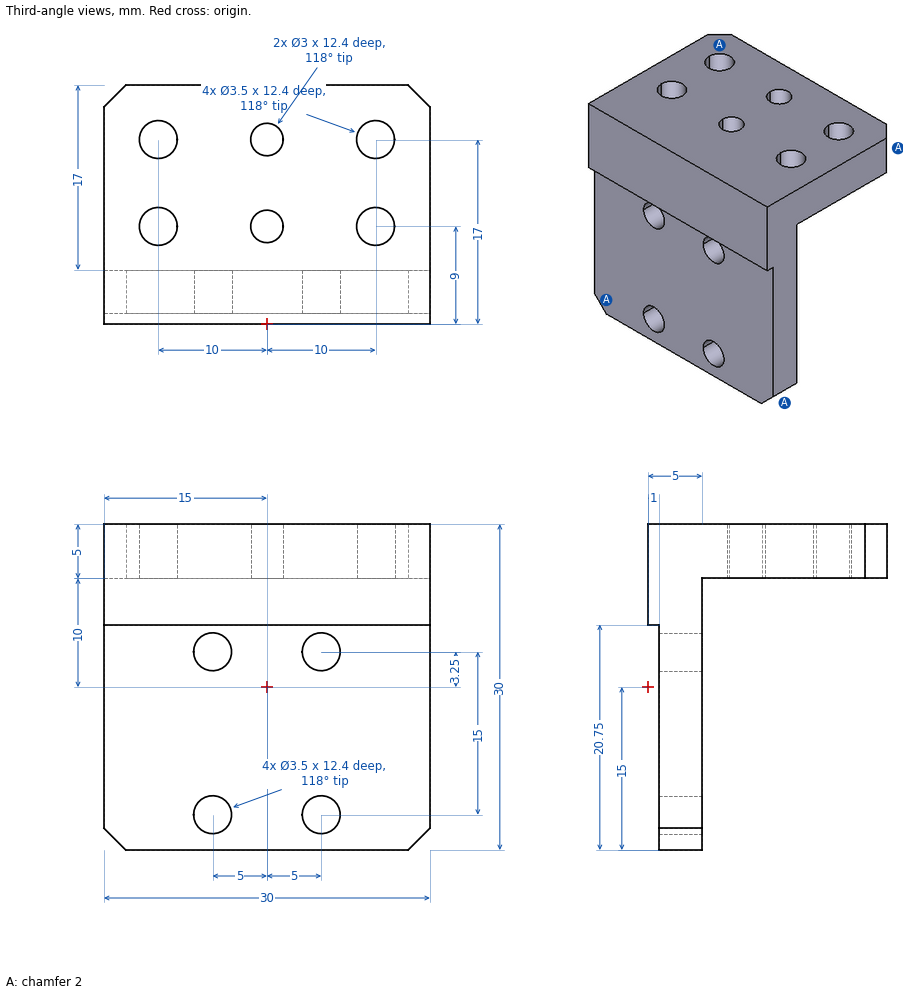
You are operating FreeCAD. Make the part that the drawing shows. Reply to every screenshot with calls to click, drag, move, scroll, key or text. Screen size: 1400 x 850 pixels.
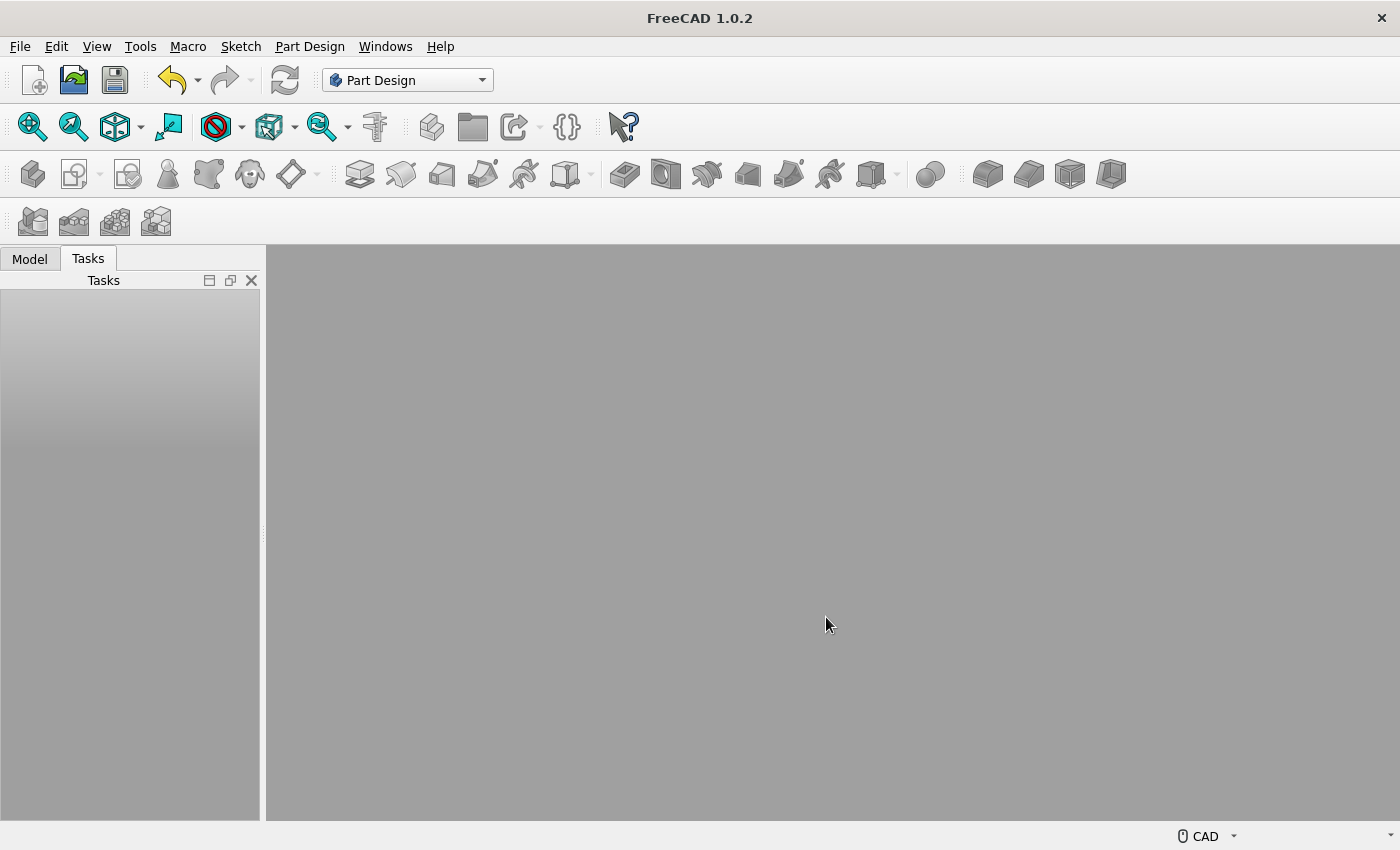
key(ctrl+n)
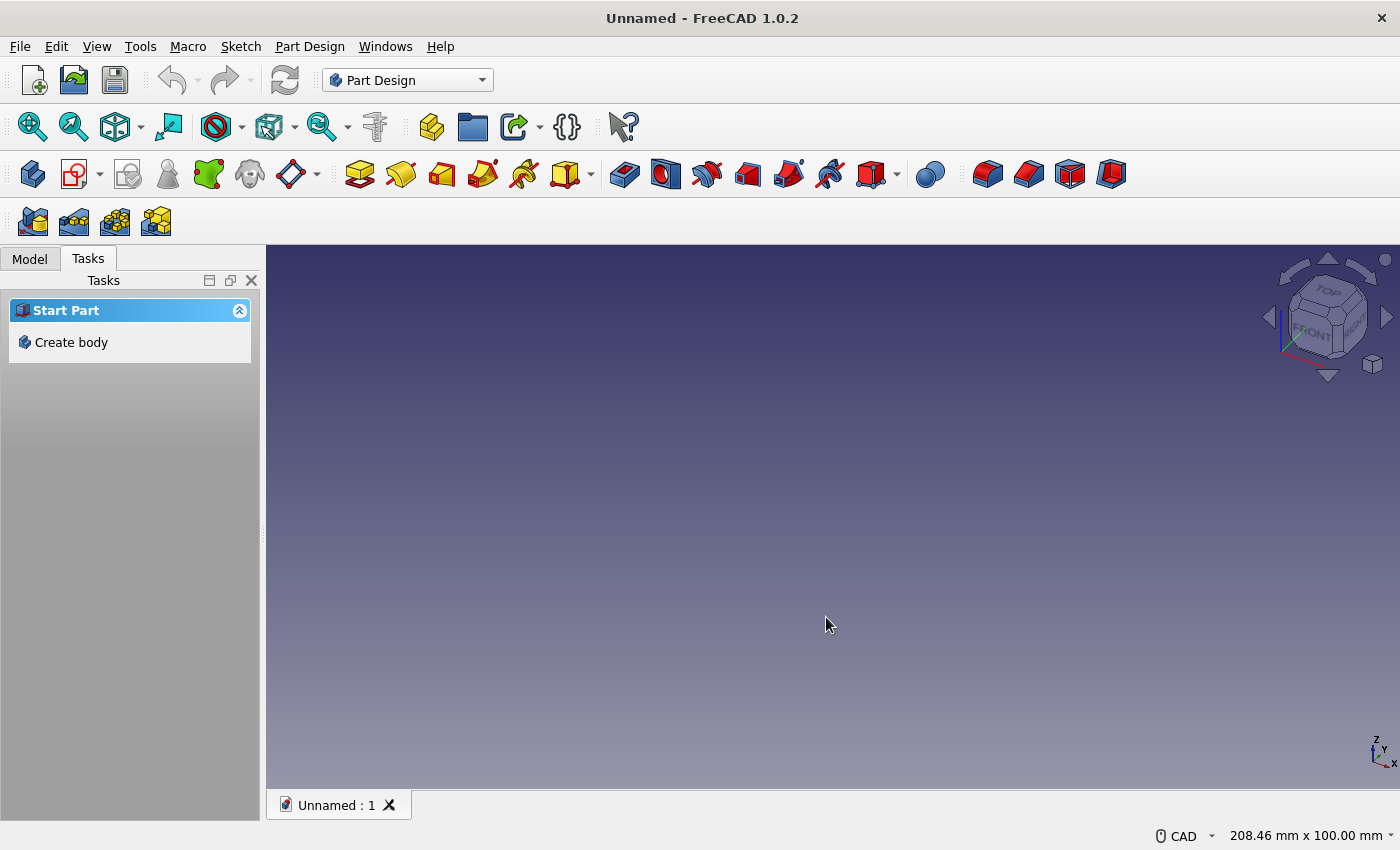
click(74, 174)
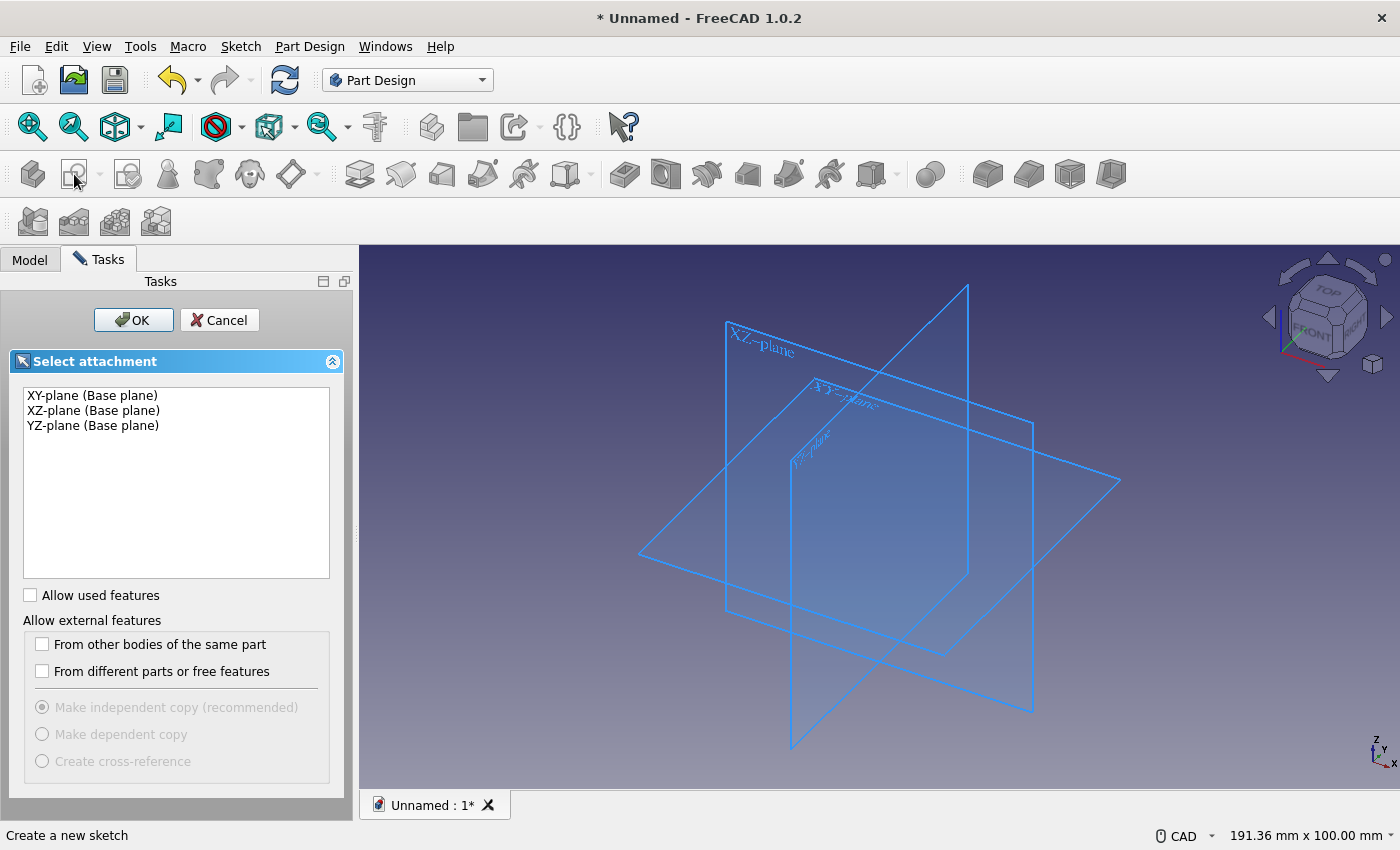
click(84, 410)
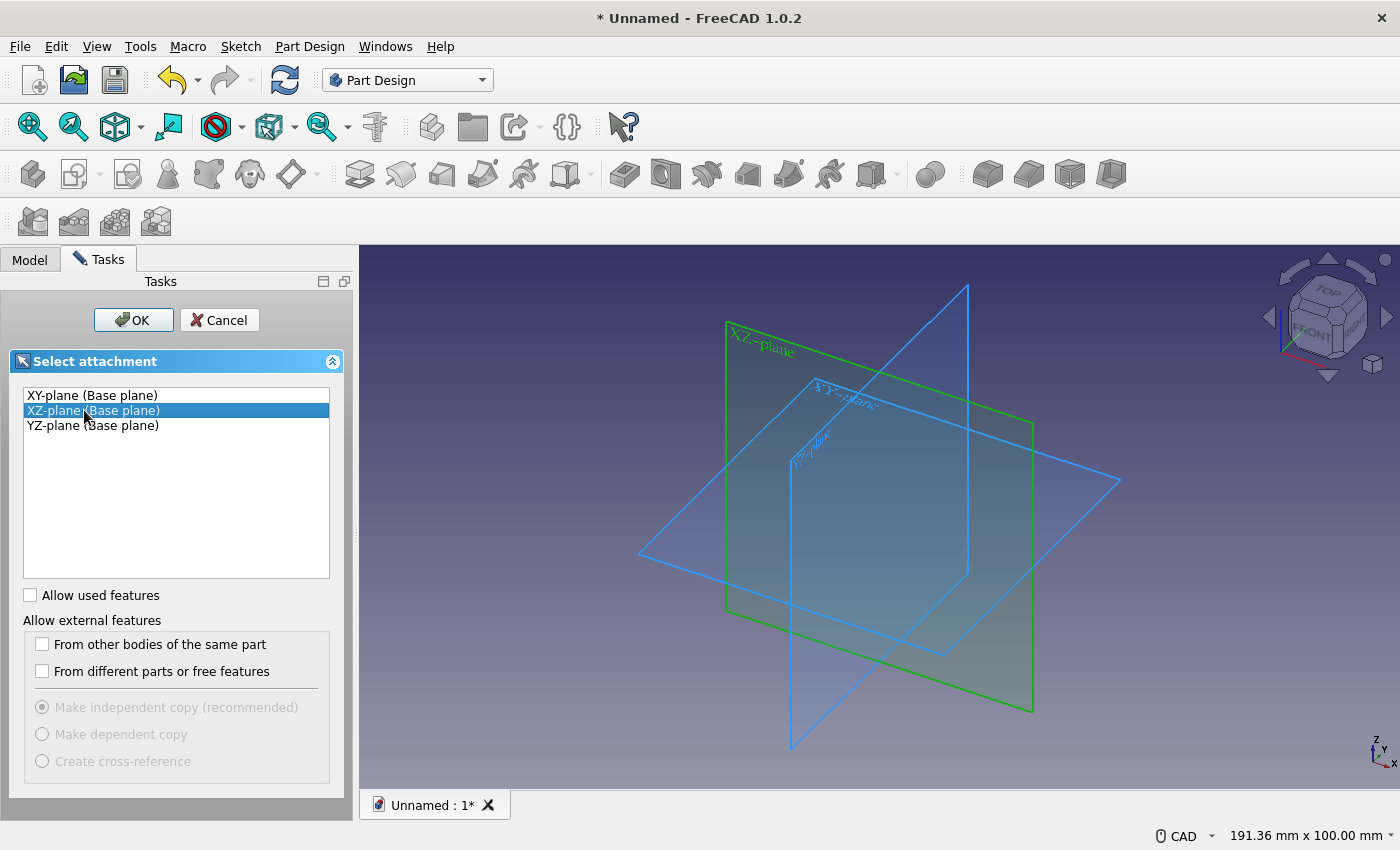
click(134, 320)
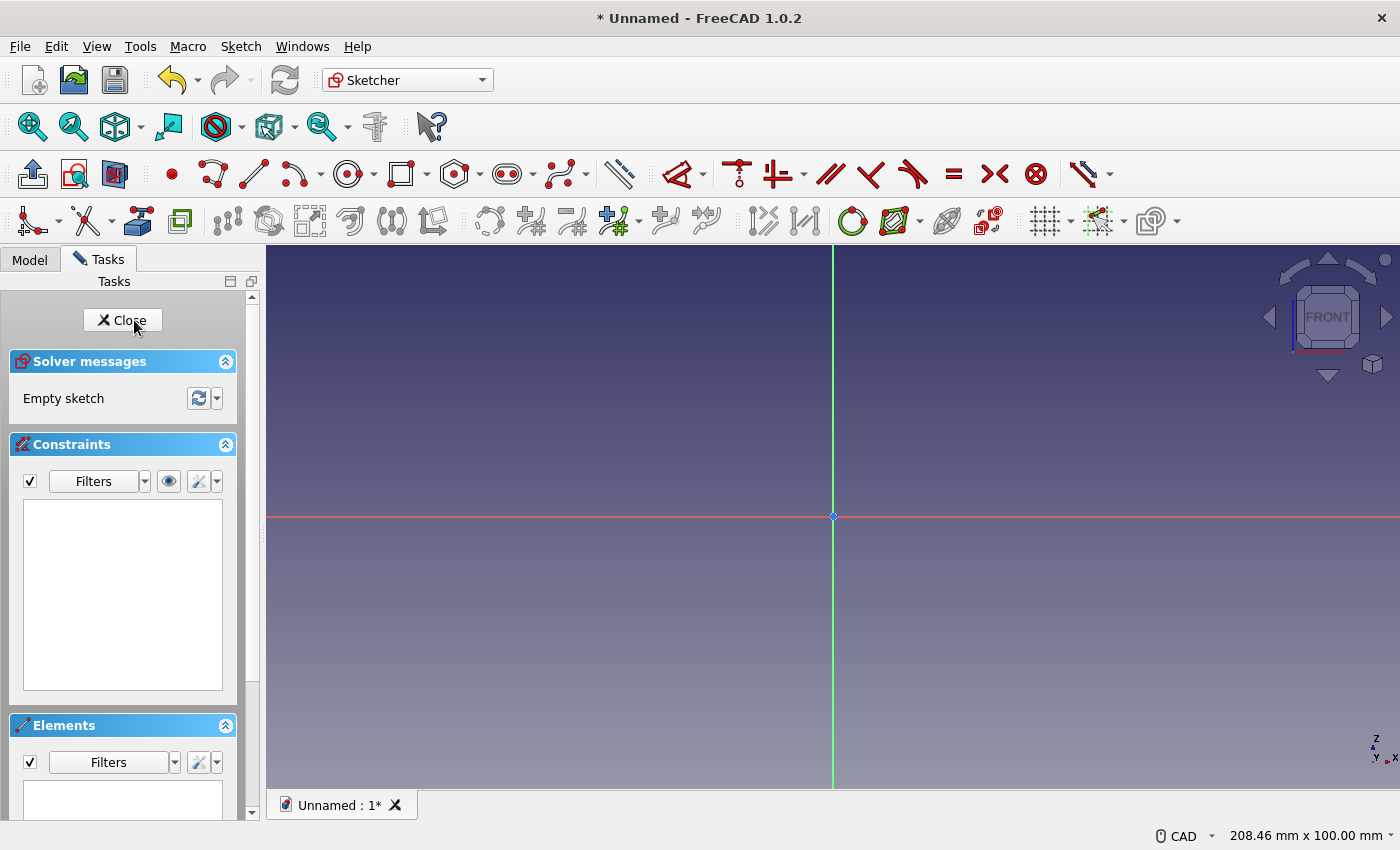
scroll(889, 517, up, 4)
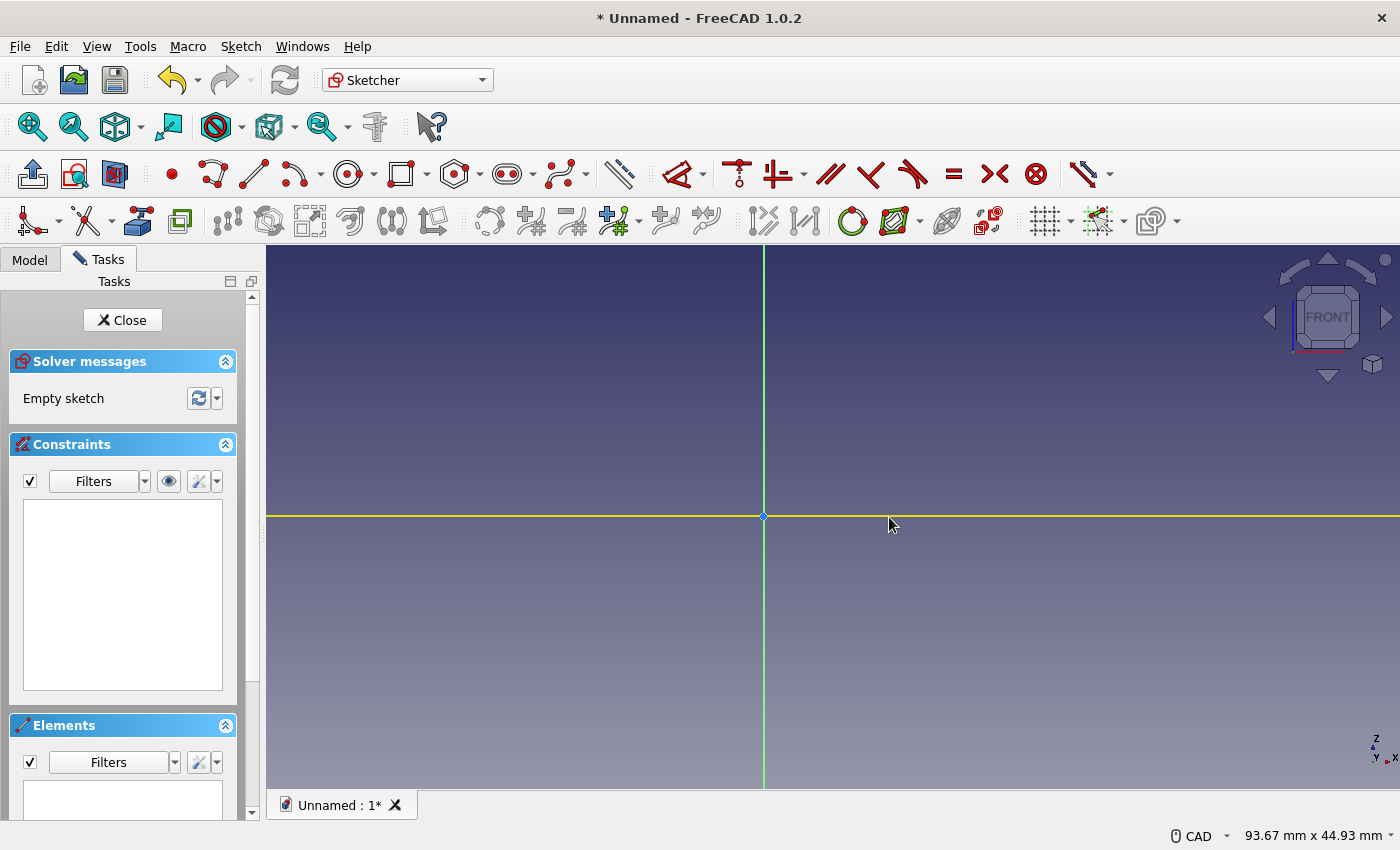
key(g)
key(v)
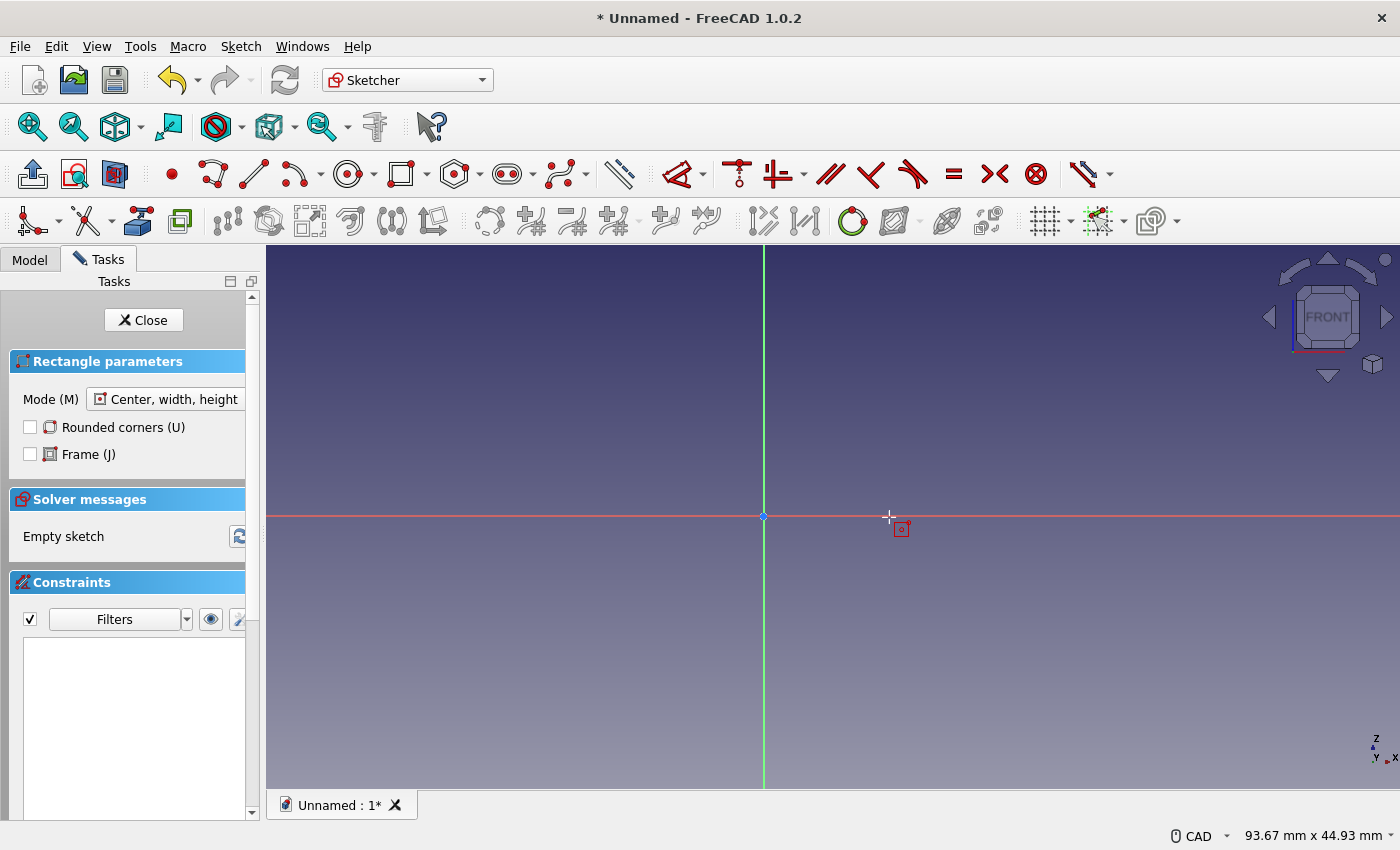
click(764, 516)
click(945, 335)
key(Escape)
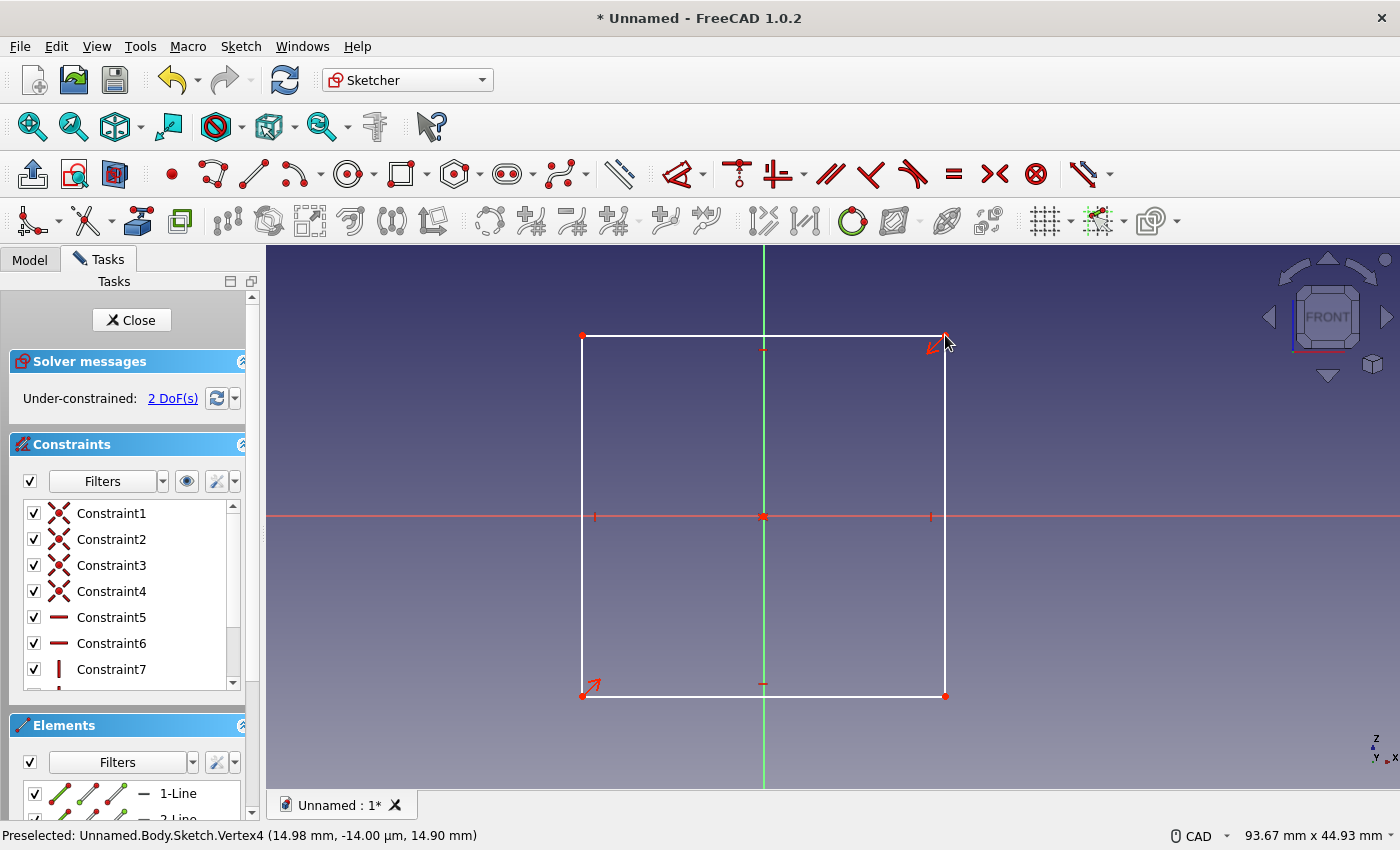
key(d)